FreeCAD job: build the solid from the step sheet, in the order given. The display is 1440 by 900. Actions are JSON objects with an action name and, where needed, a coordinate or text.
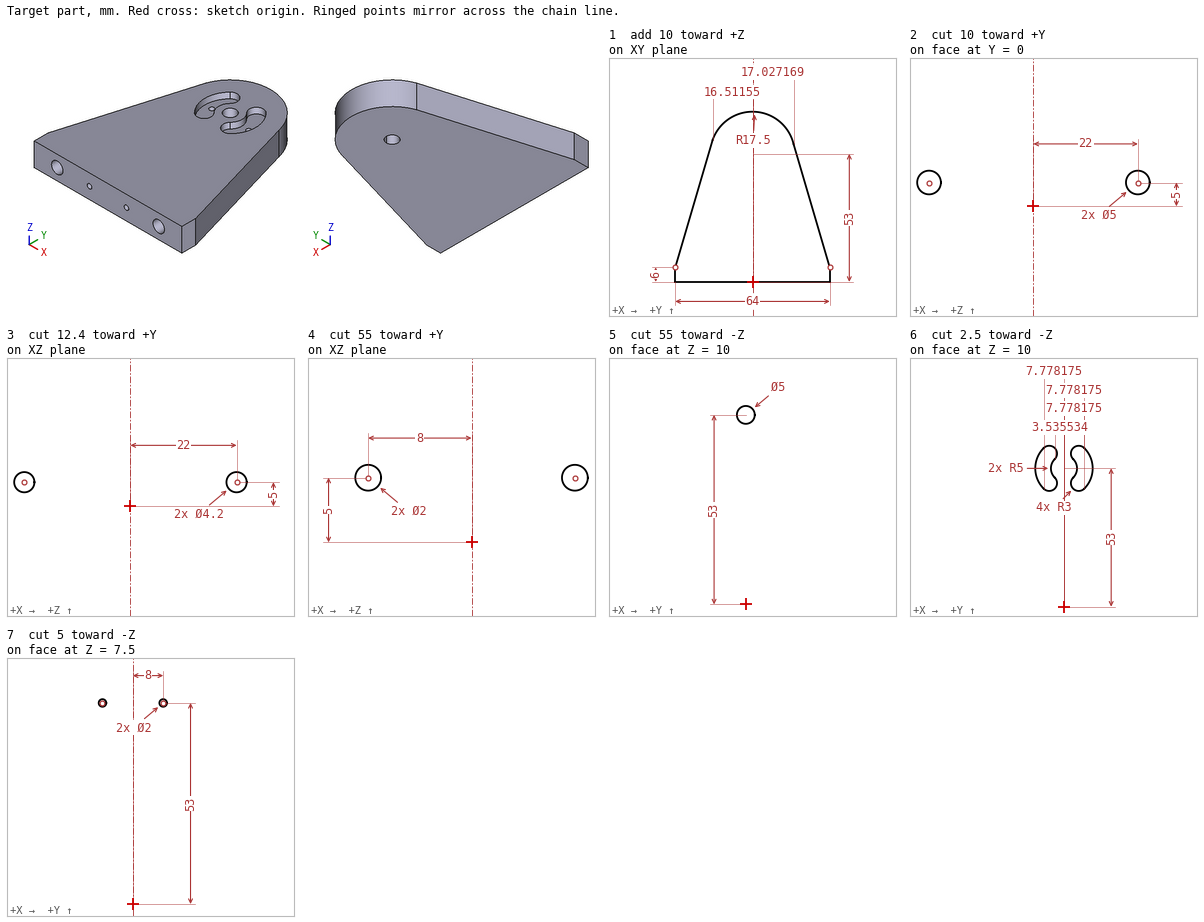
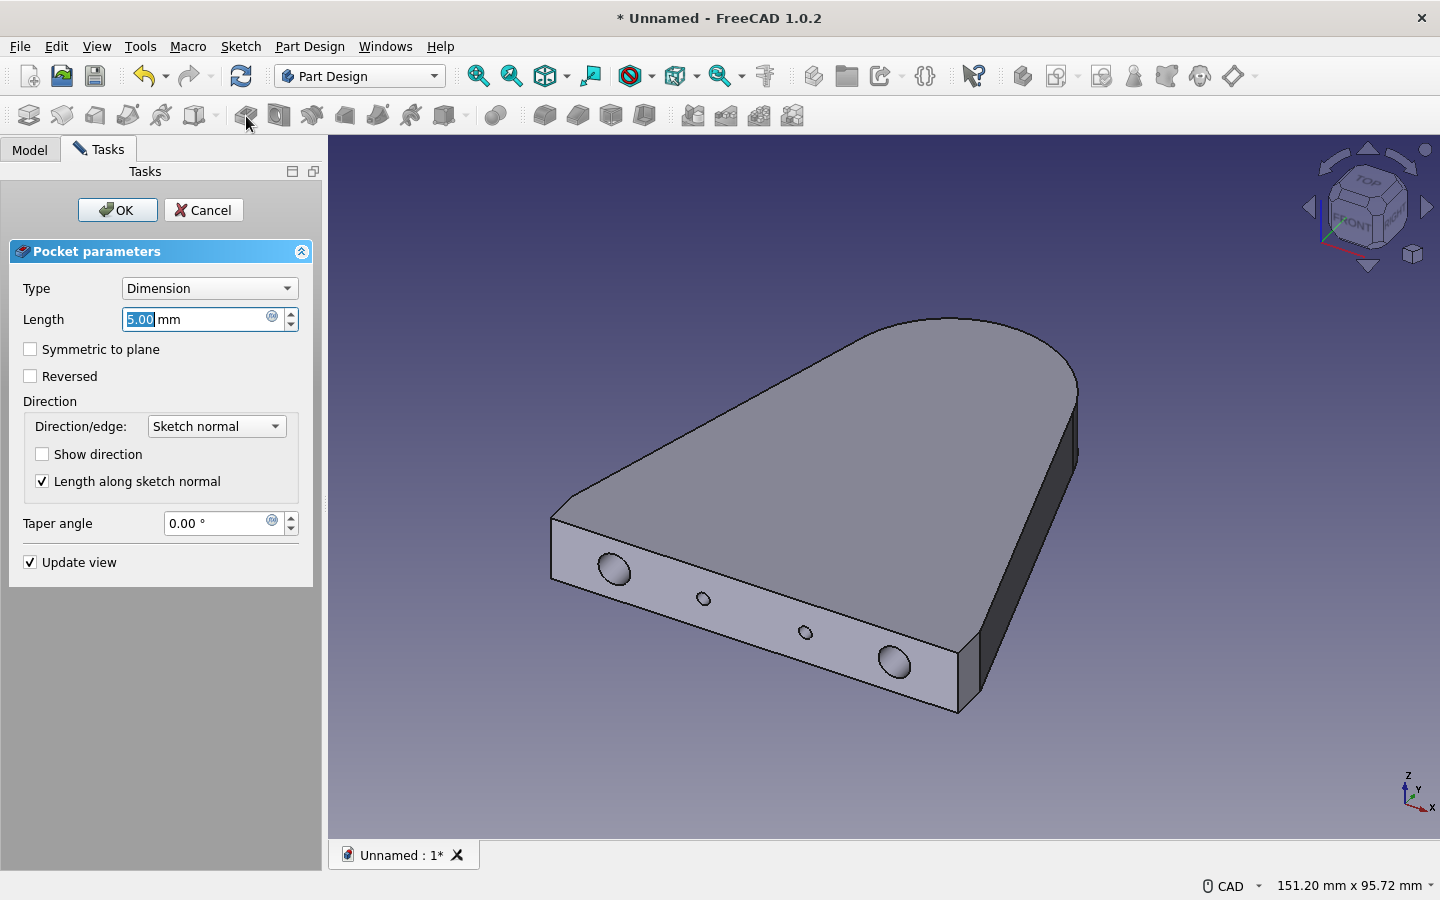
{"action": "type", "text": "55"}
{"action": "key", "text": "Tab"}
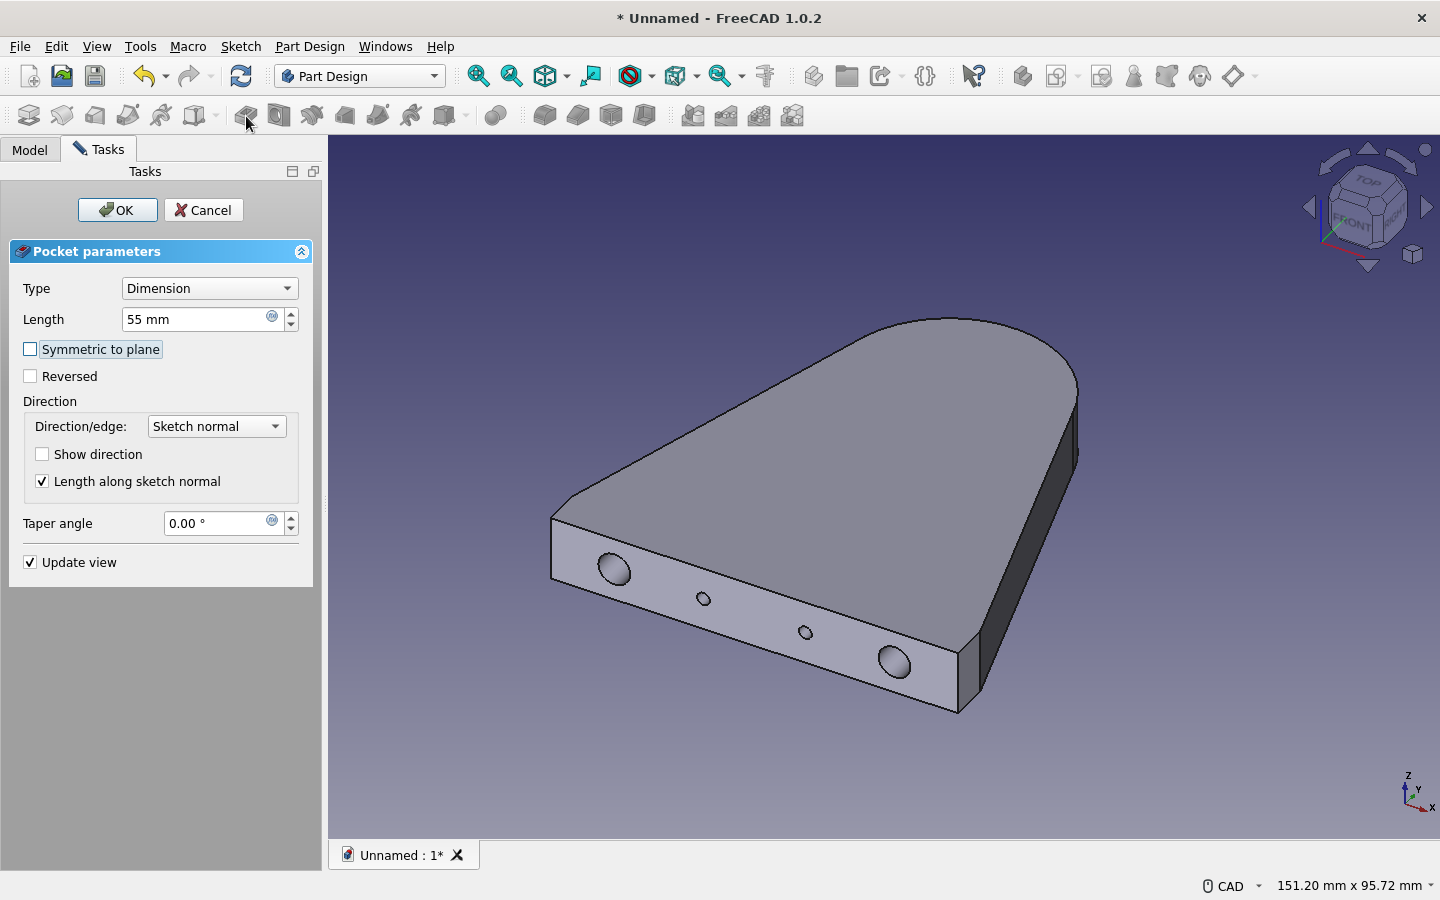
{"action": "left_click", "coordinate": [118, 210]}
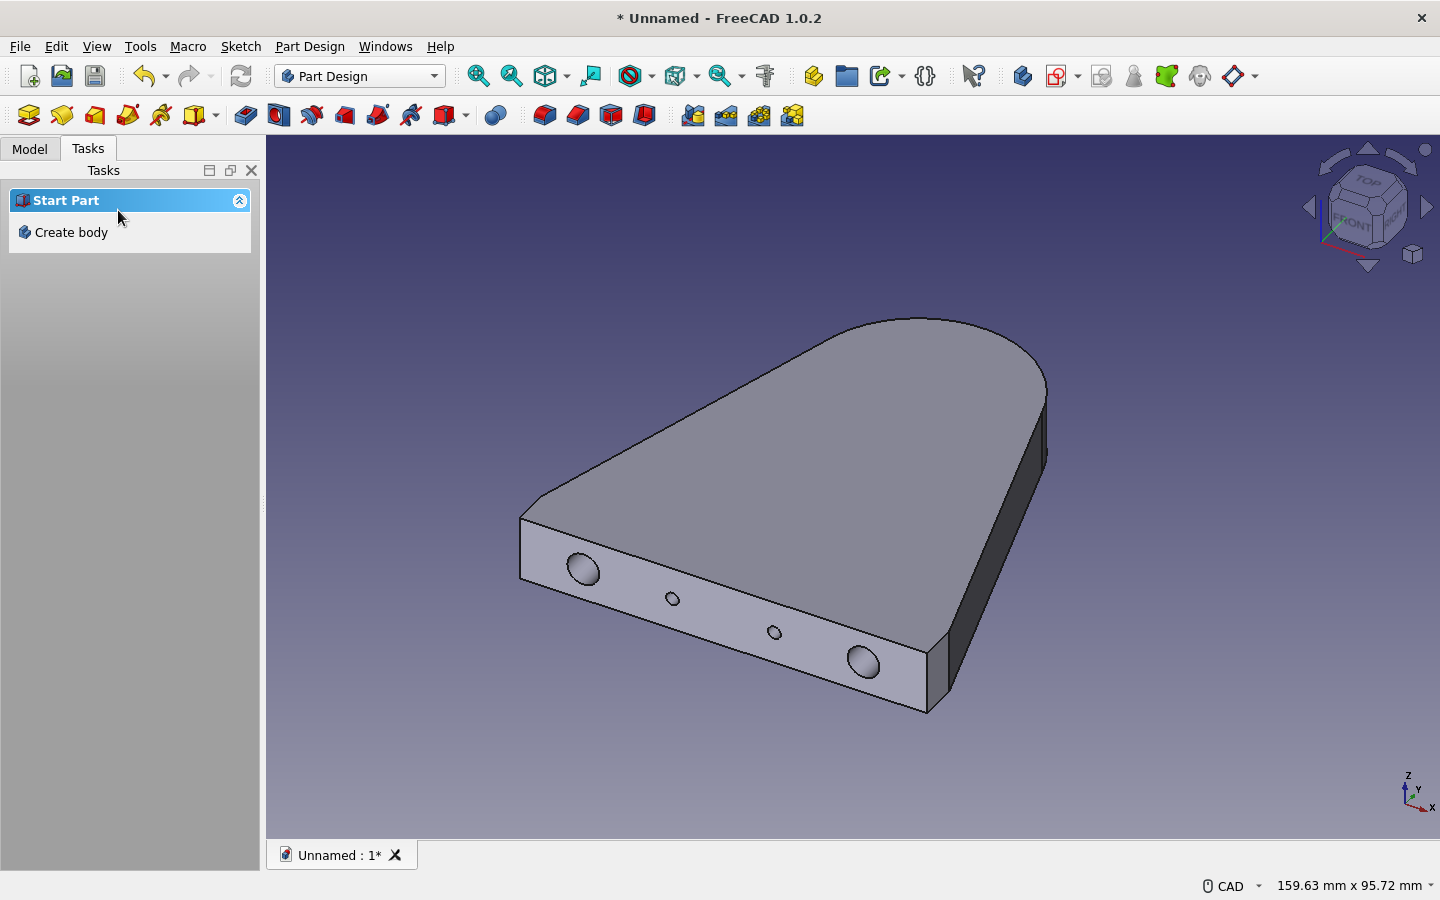
{"action": "left_click", "coordinate": [816, 493]}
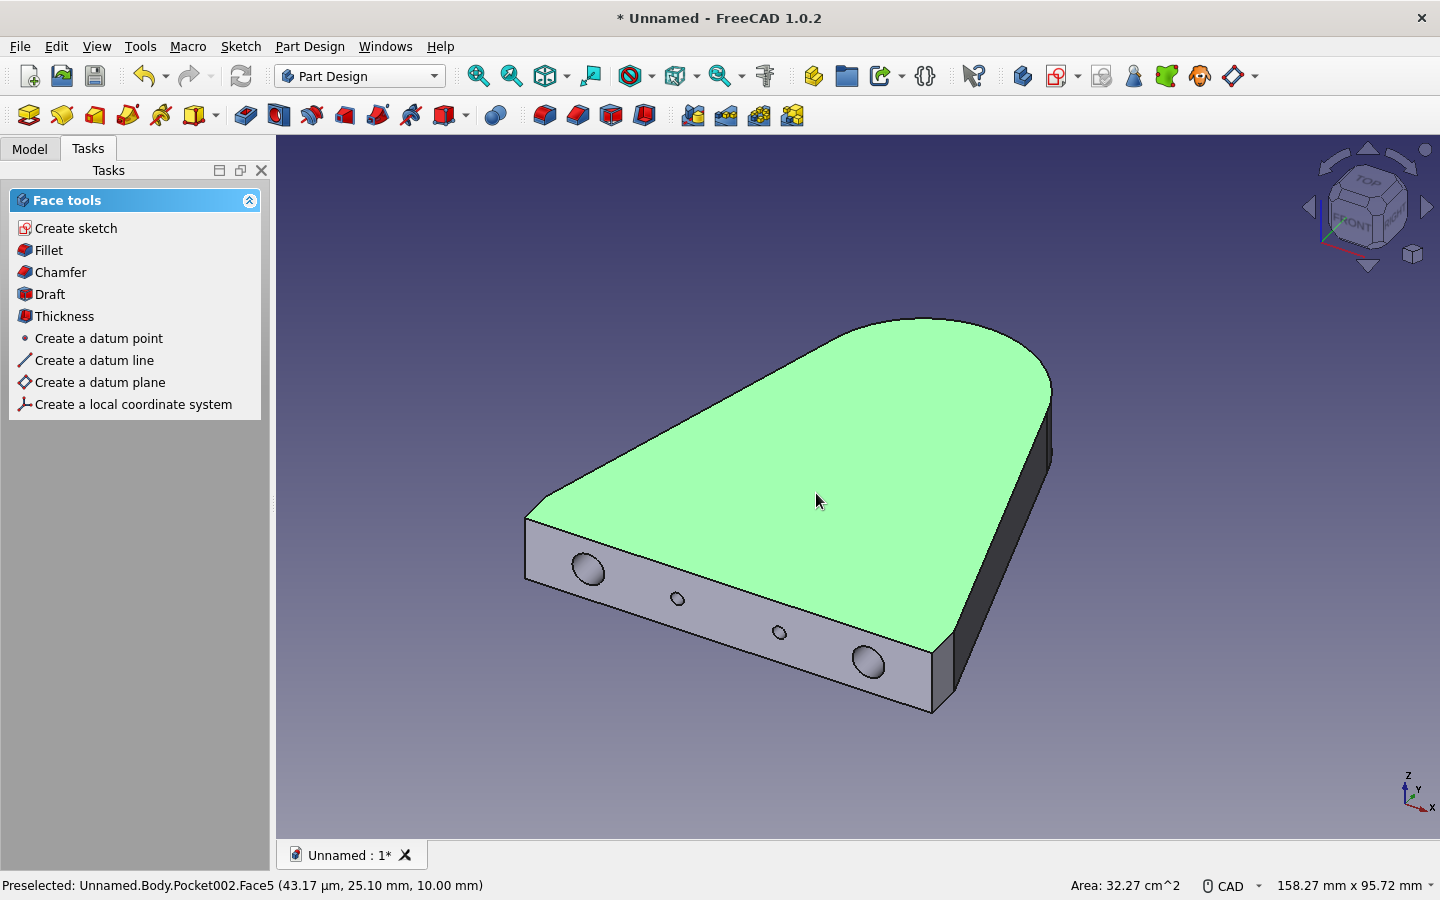
{"action": "left_click", "coordinate": [1056, 76]}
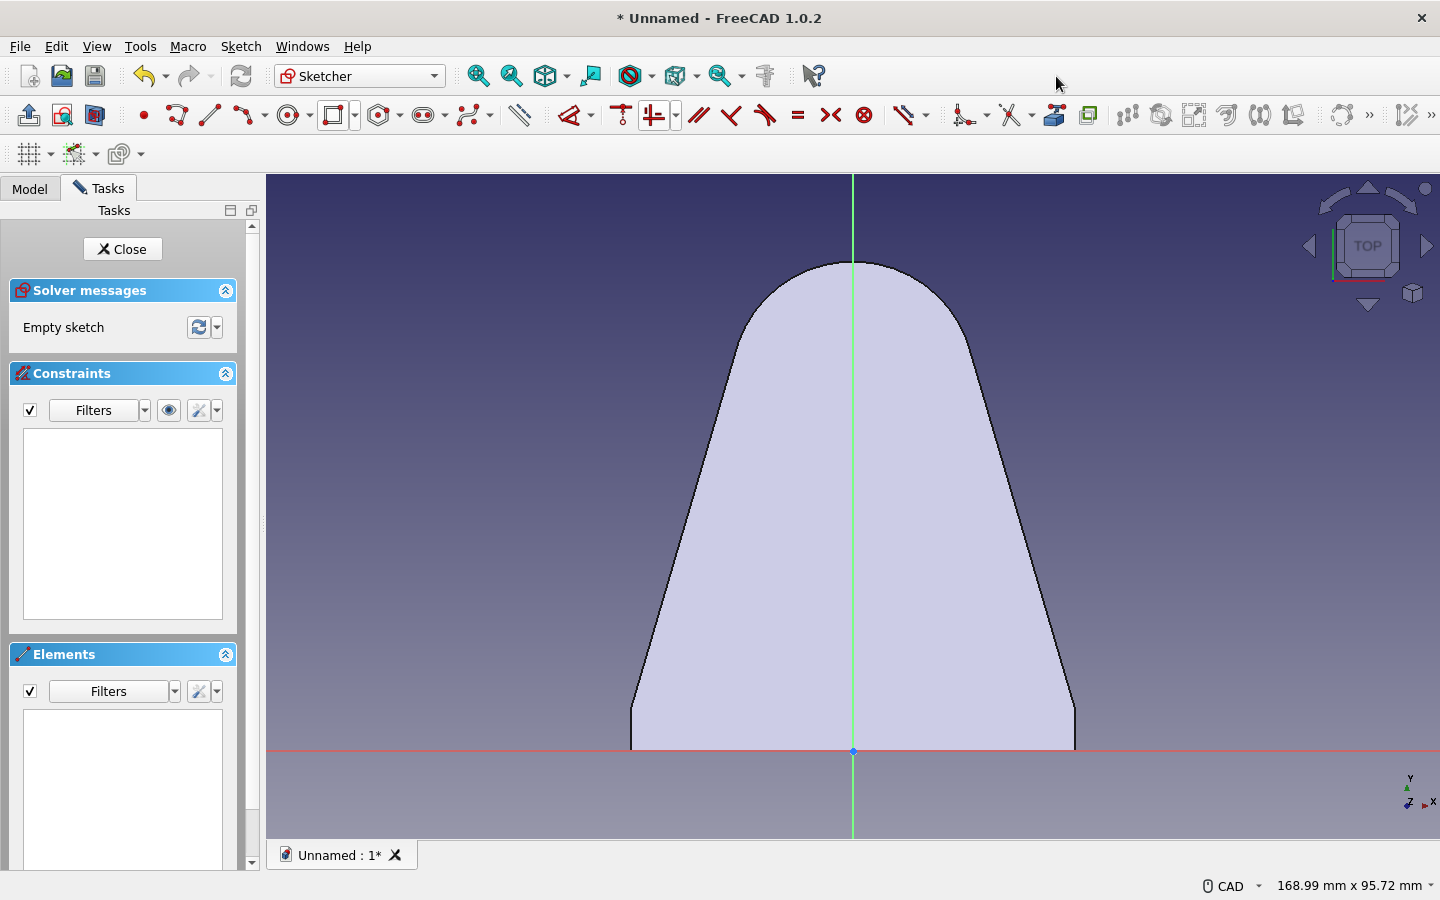
{"action": "scroll", "coordinate": [858, 373], "scroll_direction": "up", "scroll_amount": 13}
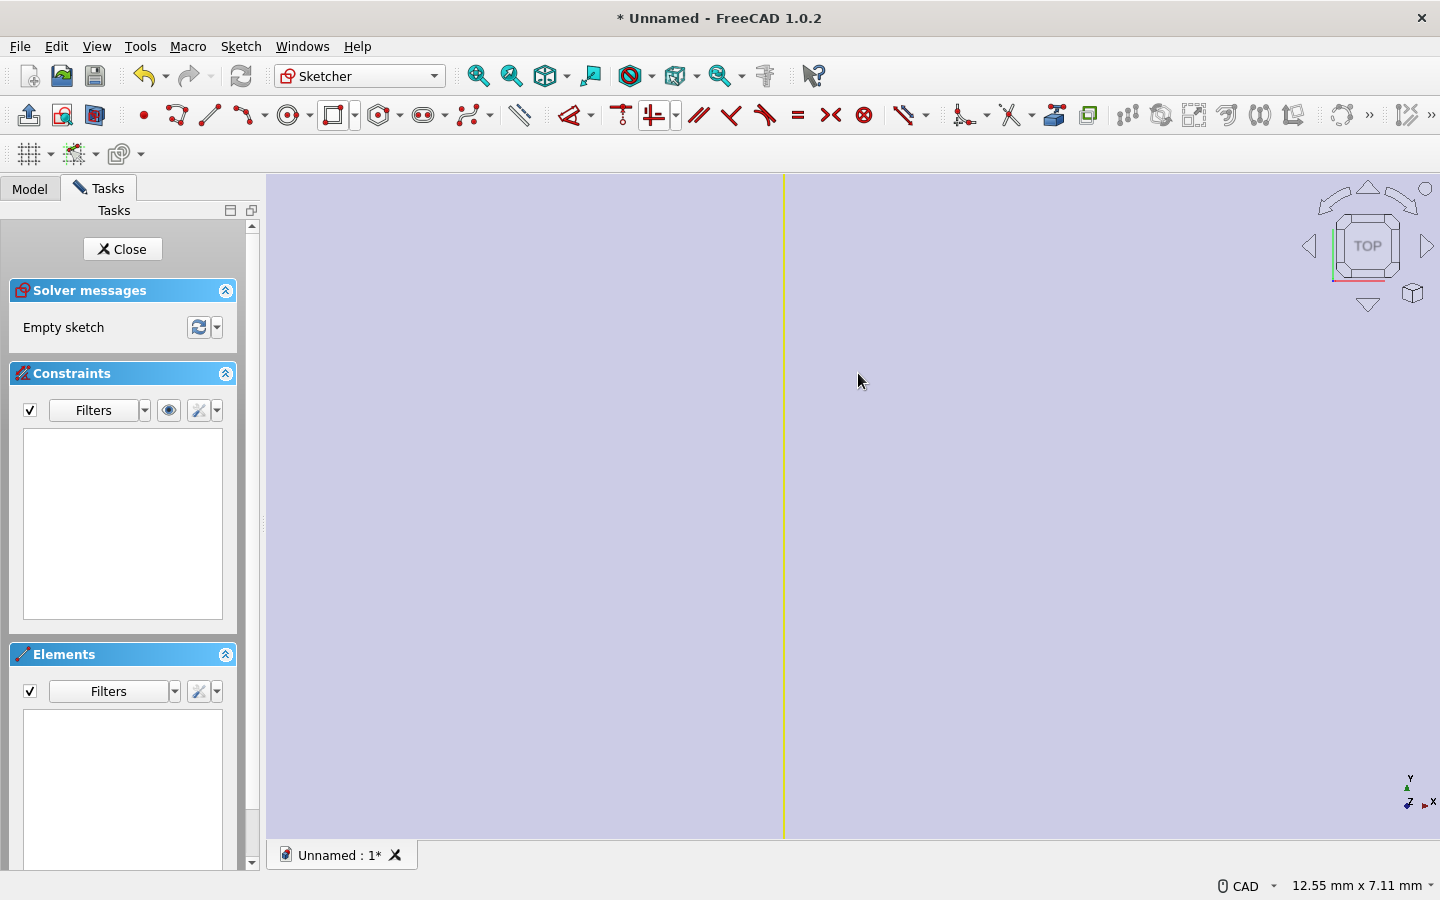
{"action": "left_click", "coordinate": [288, 116]}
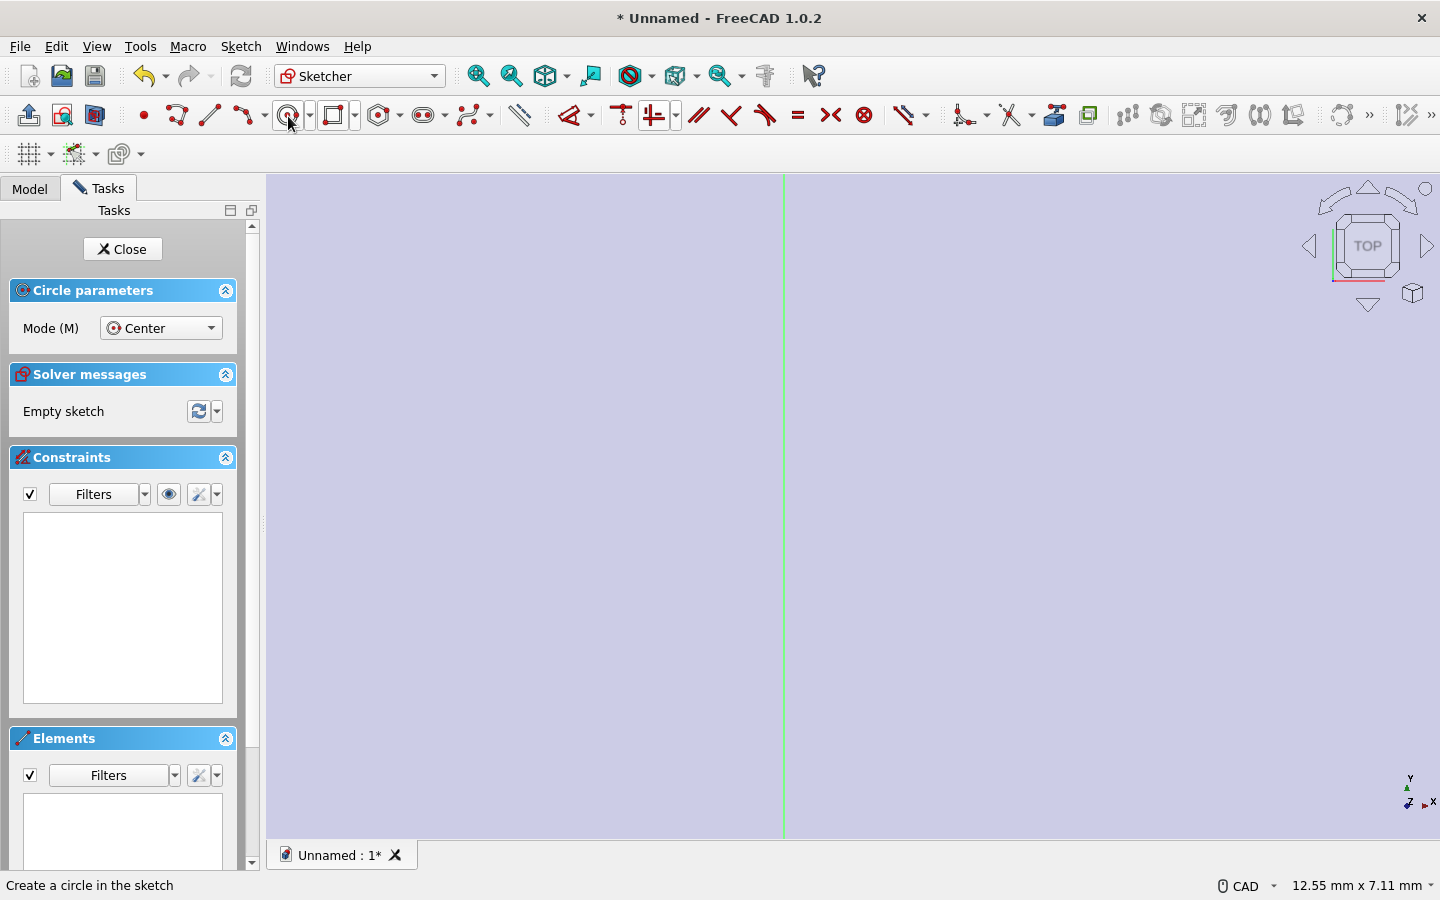
{"action": "left_click", "coordinate": [784, 505]}
{"action": "mouse_move", "coordinate": [950, 340]}